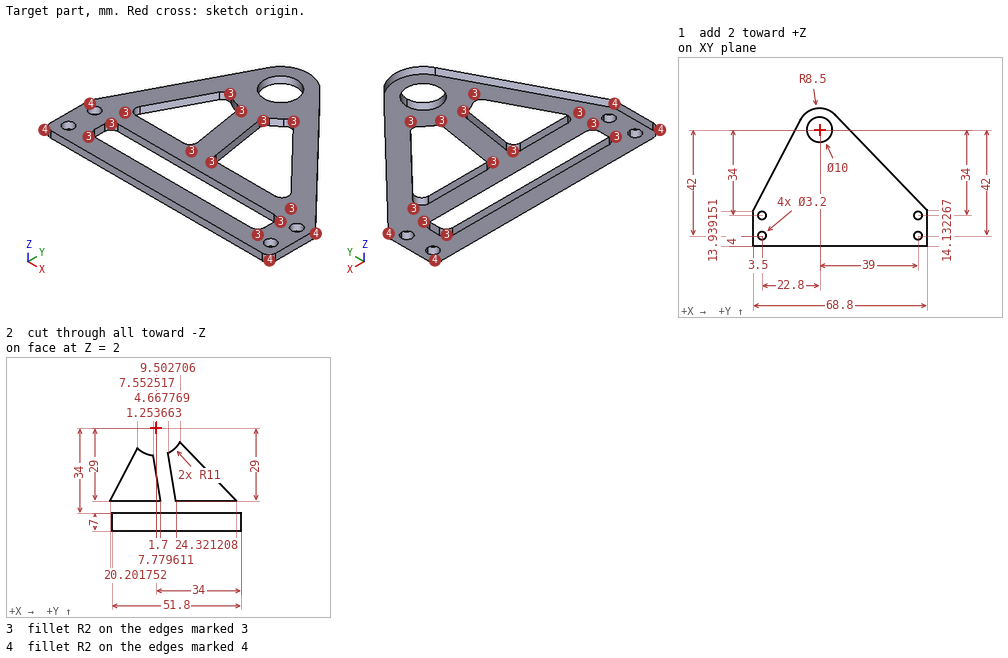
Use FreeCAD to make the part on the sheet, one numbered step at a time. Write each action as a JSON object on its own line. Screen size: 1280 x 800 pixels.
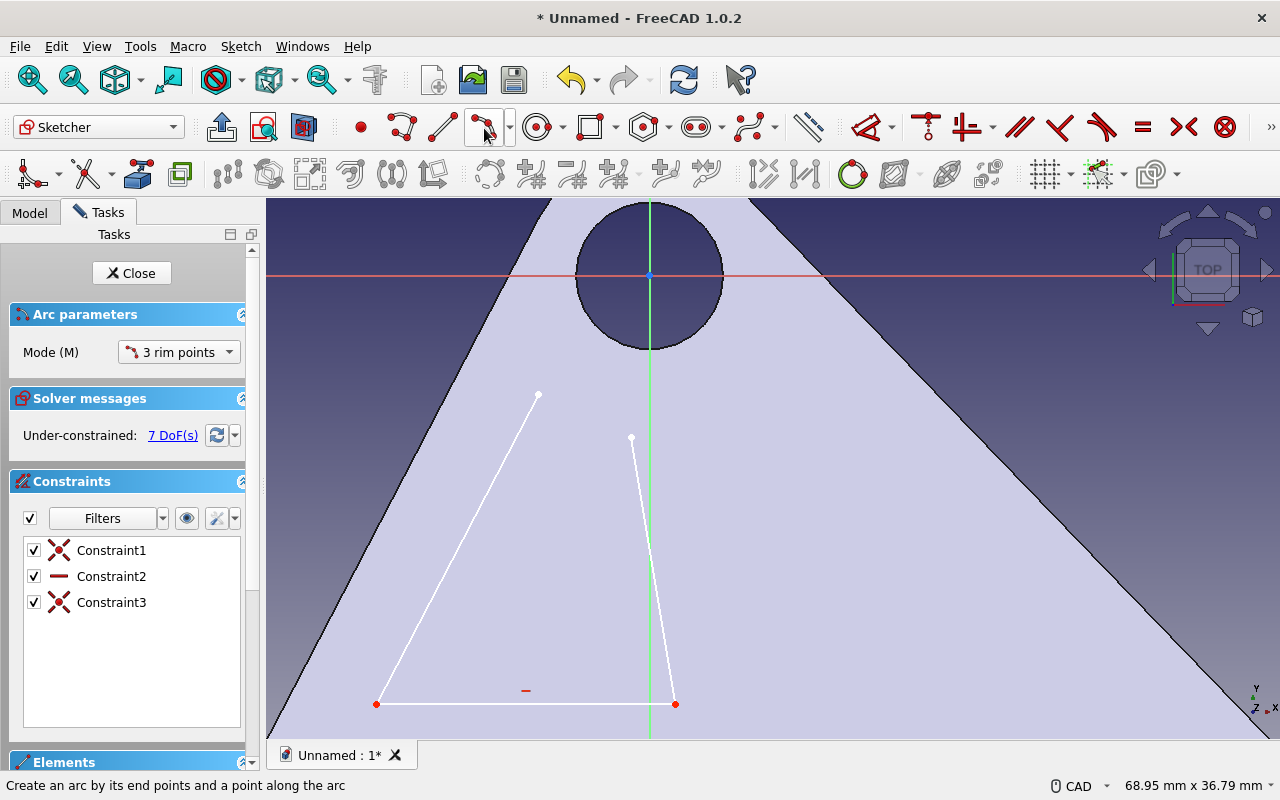
{"action": "left_click", "coordinate": [631, 438]}
{"action": "left_click", "coordinate": [539, 395]}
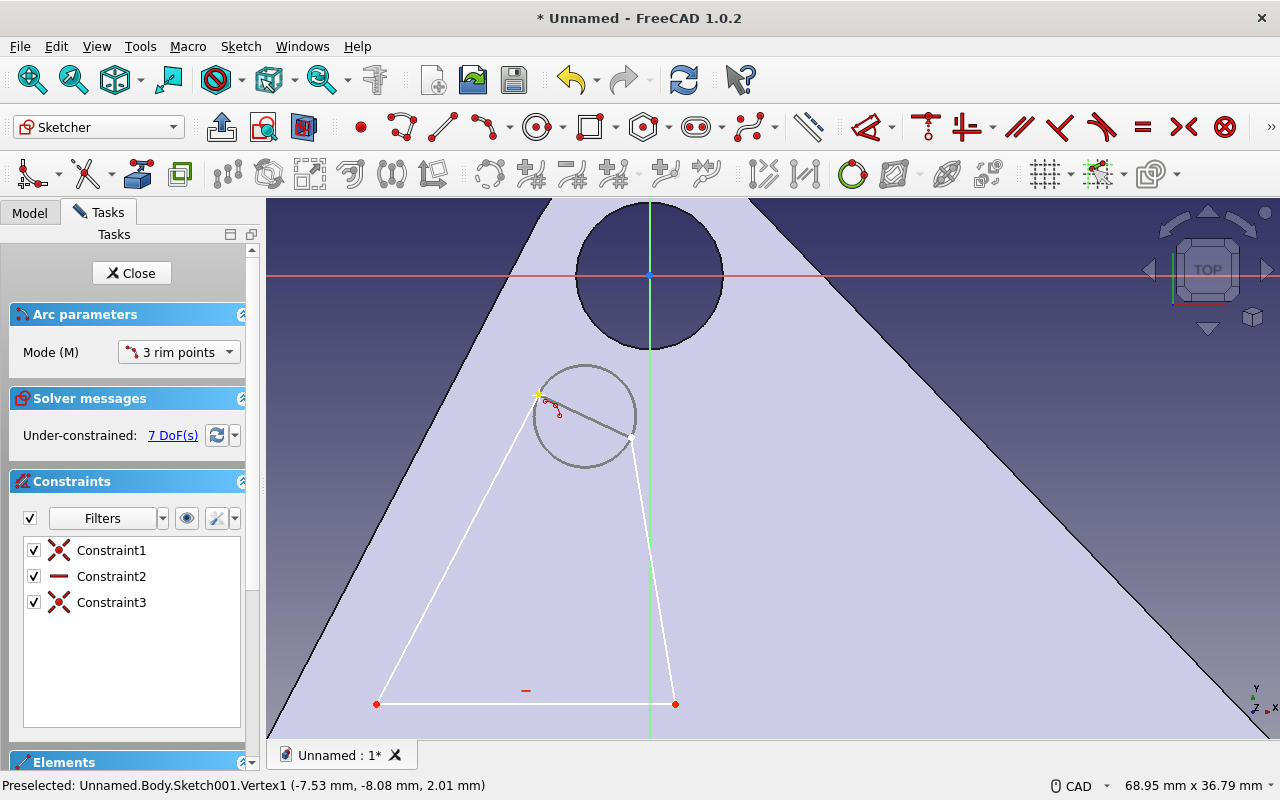
{"action": "scroll", "coordinate": [581, 423], "scroll_direction": "up", "scroll_amount": 4}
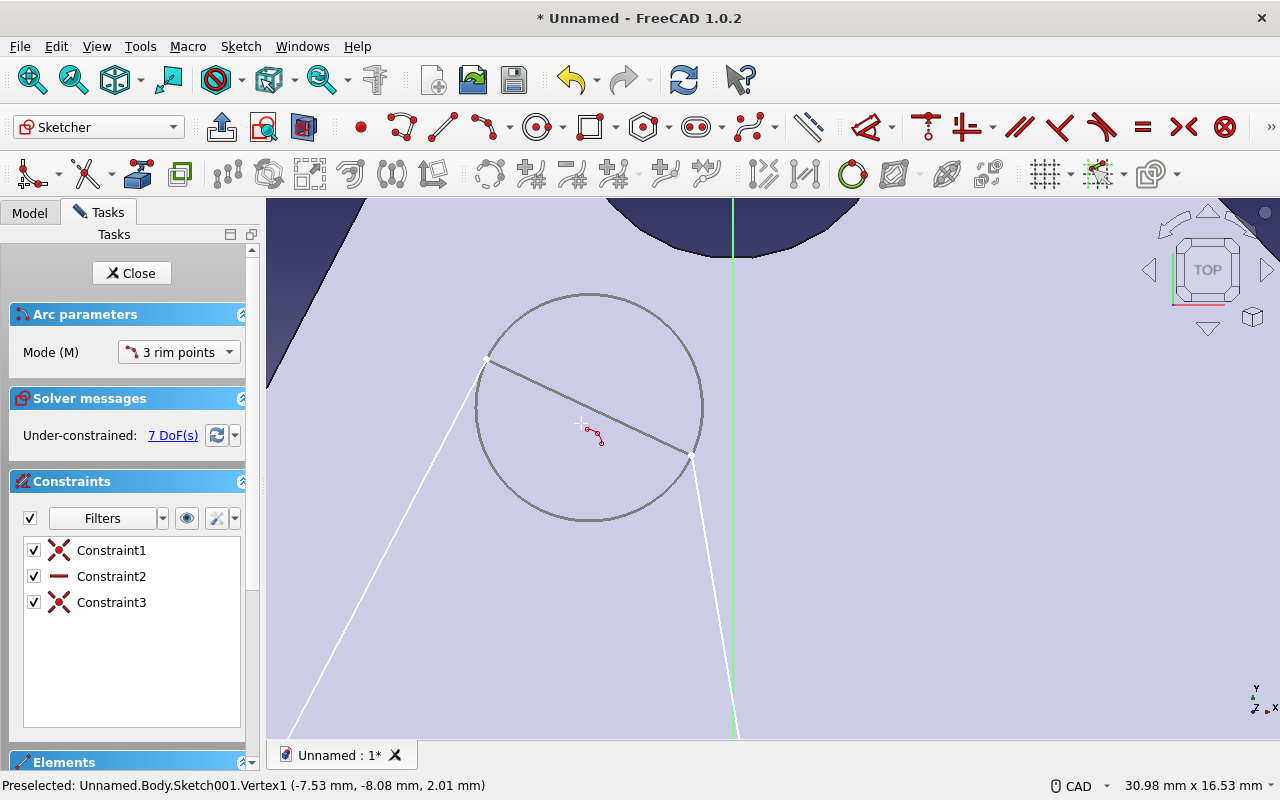
{"action": "left_click", "coordinate": [581, 421]}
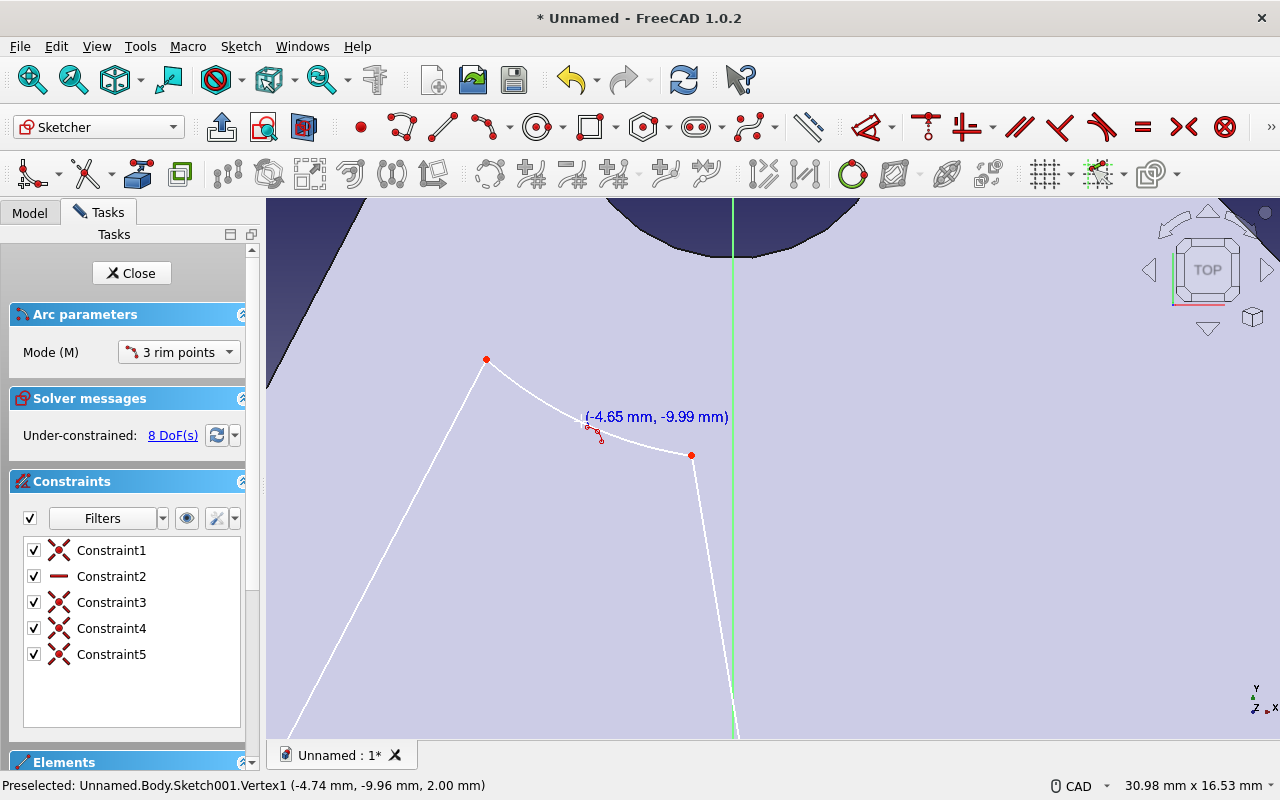
{"action": "left_click", "coordinate": [402, 128]}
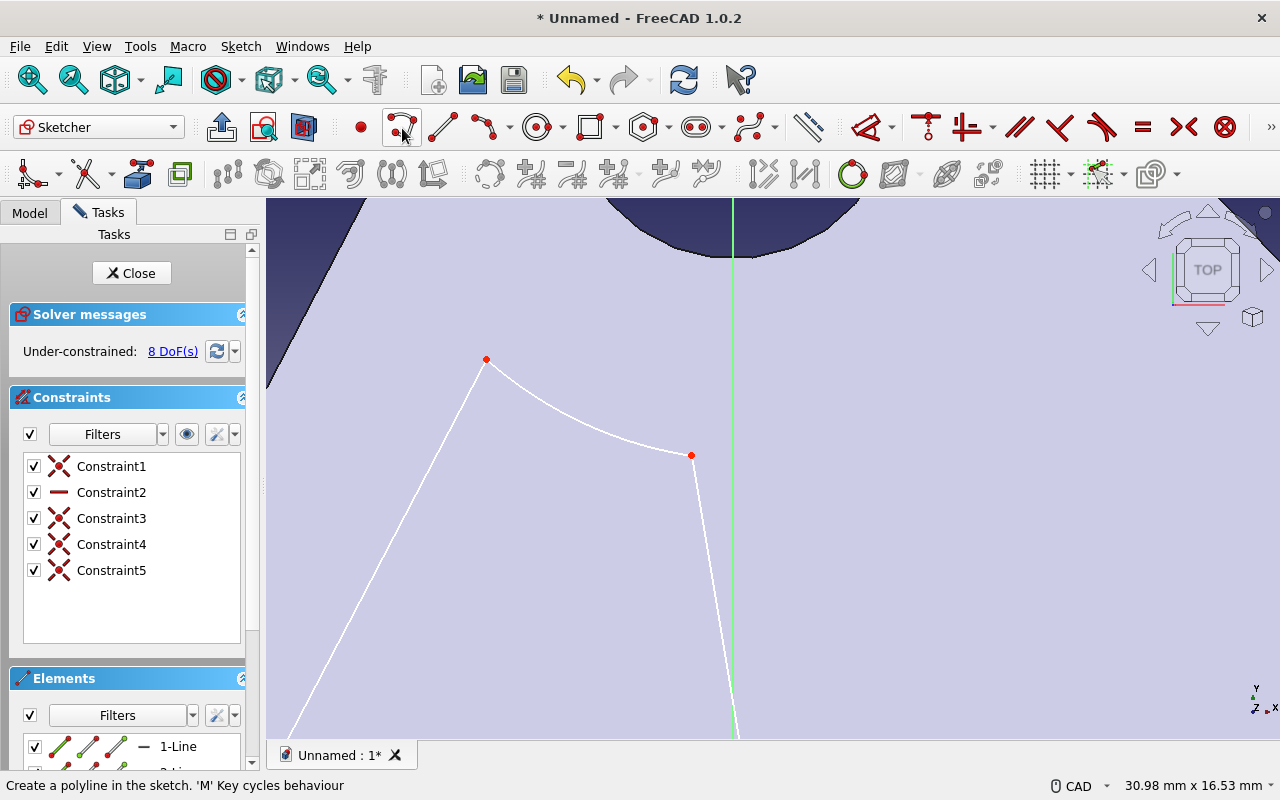
{"action": "scroll", "coordinate": [612, 371], "scroll_direction": "down", "scroll_amount": 7}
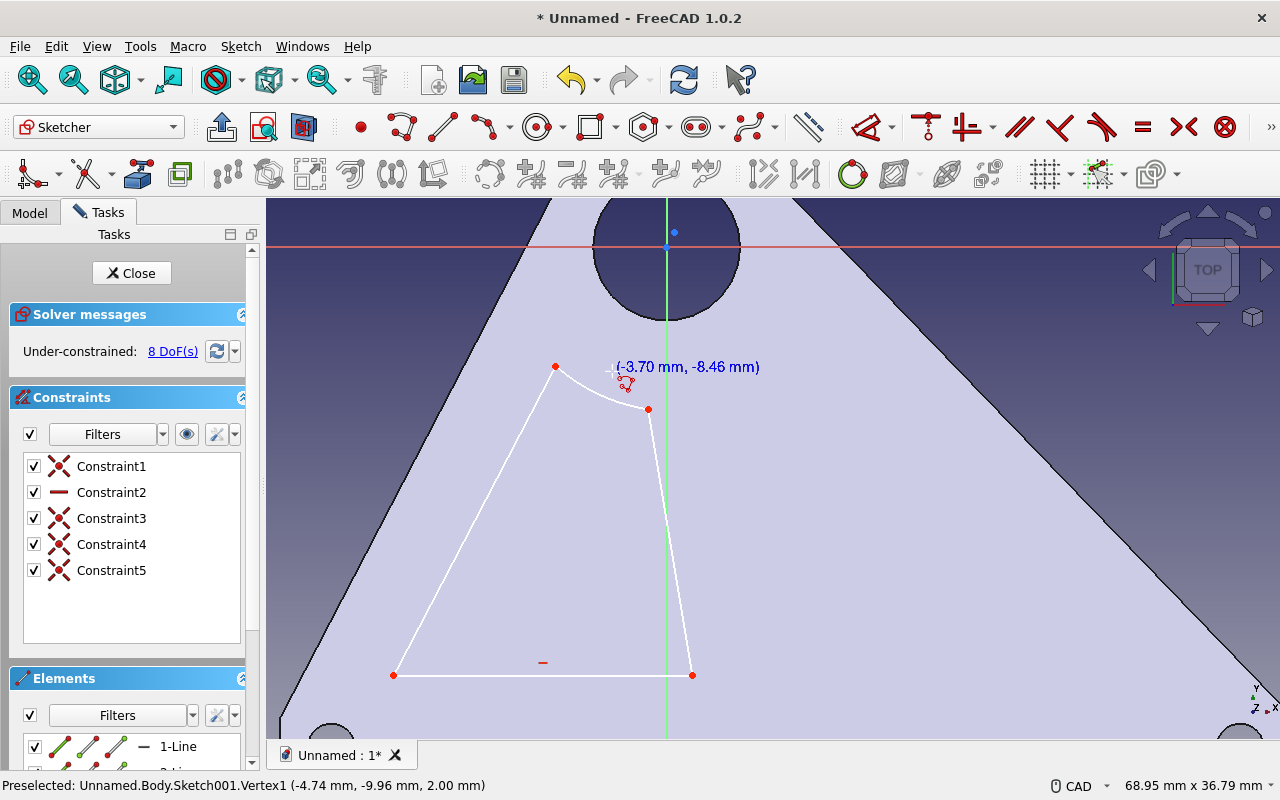
{"action": "left_click", "coordinate": [680, 384]}
{"action": "left_click", "coordinate": [705, 537]}
{"action": "left_click", "coordinate": [901, 537]}
{"action": "left_click", "coordinate": [719, 348]}
{"action": "right_click", "coordinate": [719, 348]}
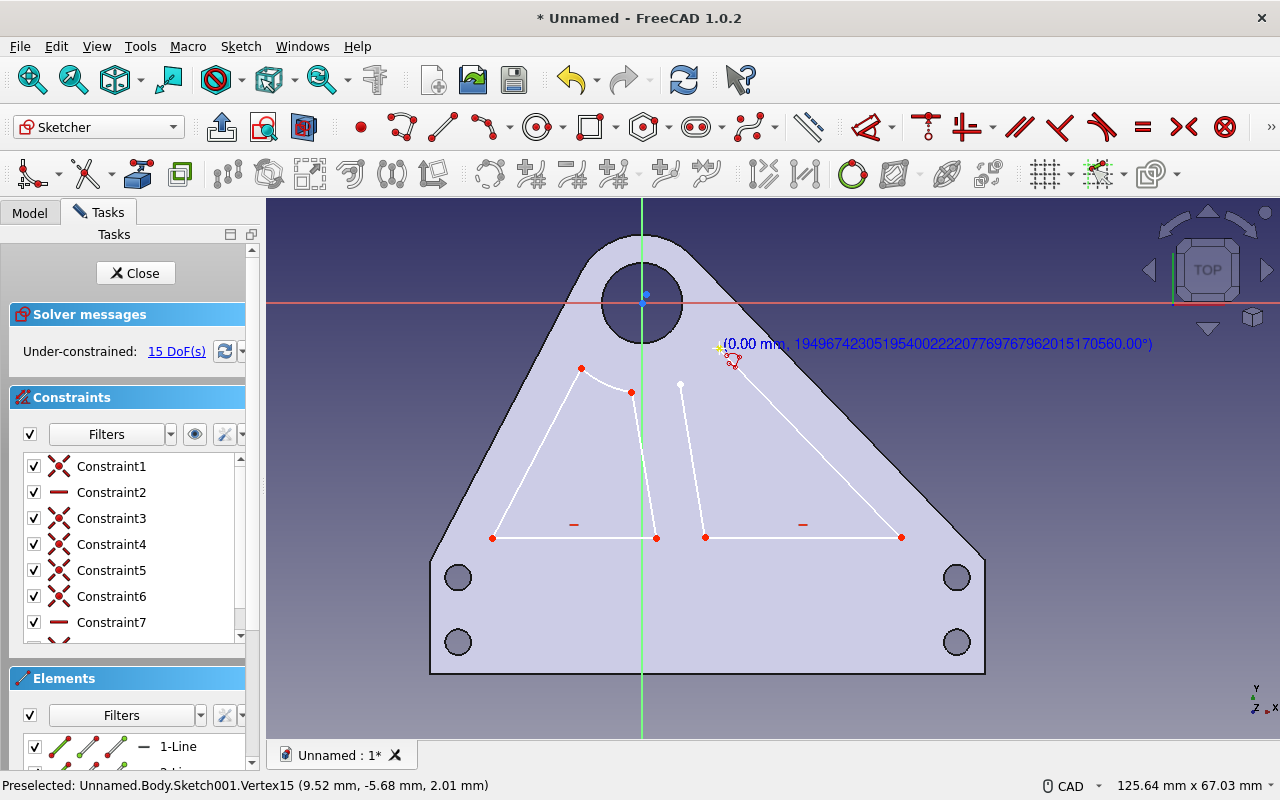
{"action": "key", "text": "g 3 a"}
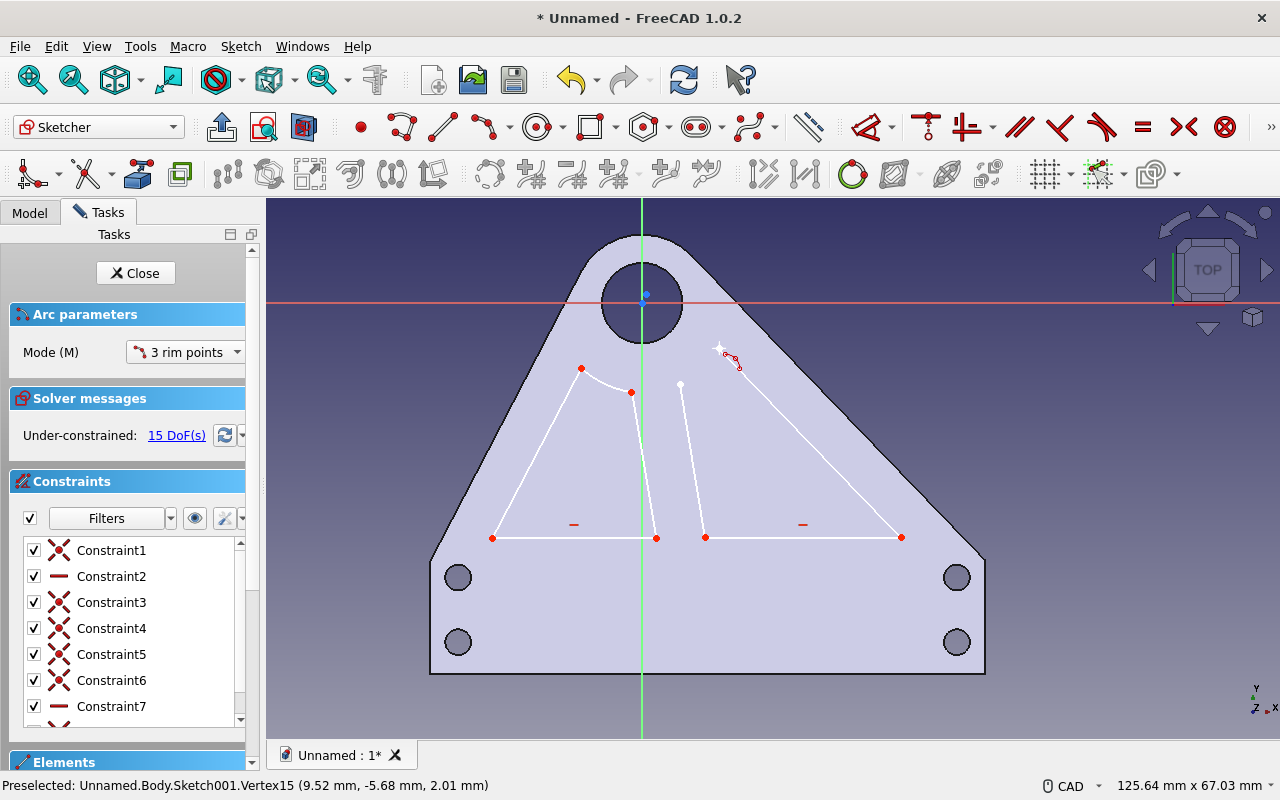
{"action": "left_click", "coordinate": [719, 349]}
{"action": "left_click", "coordinate": [680, 385]}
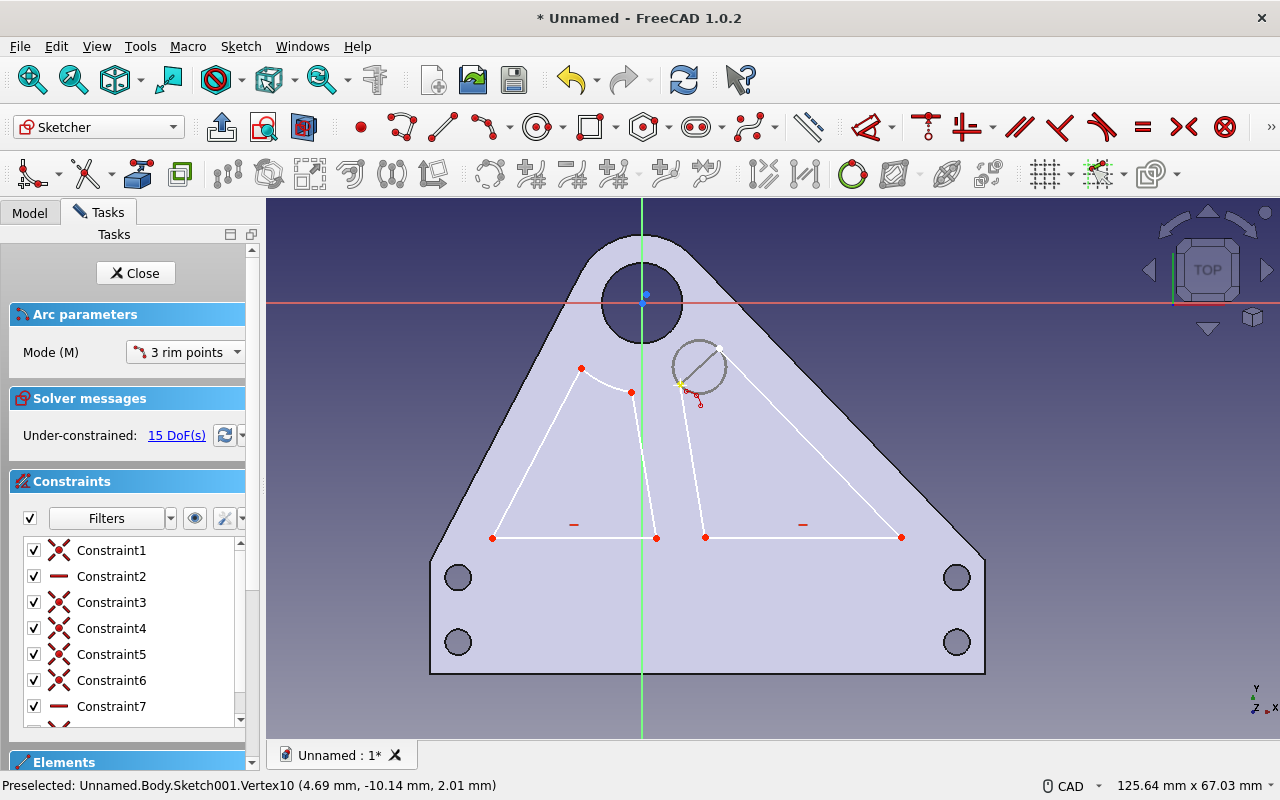
{"action": "scroll", "coordinate": [702, 369], "scroll_direction": "up", "scroll_amount": 7}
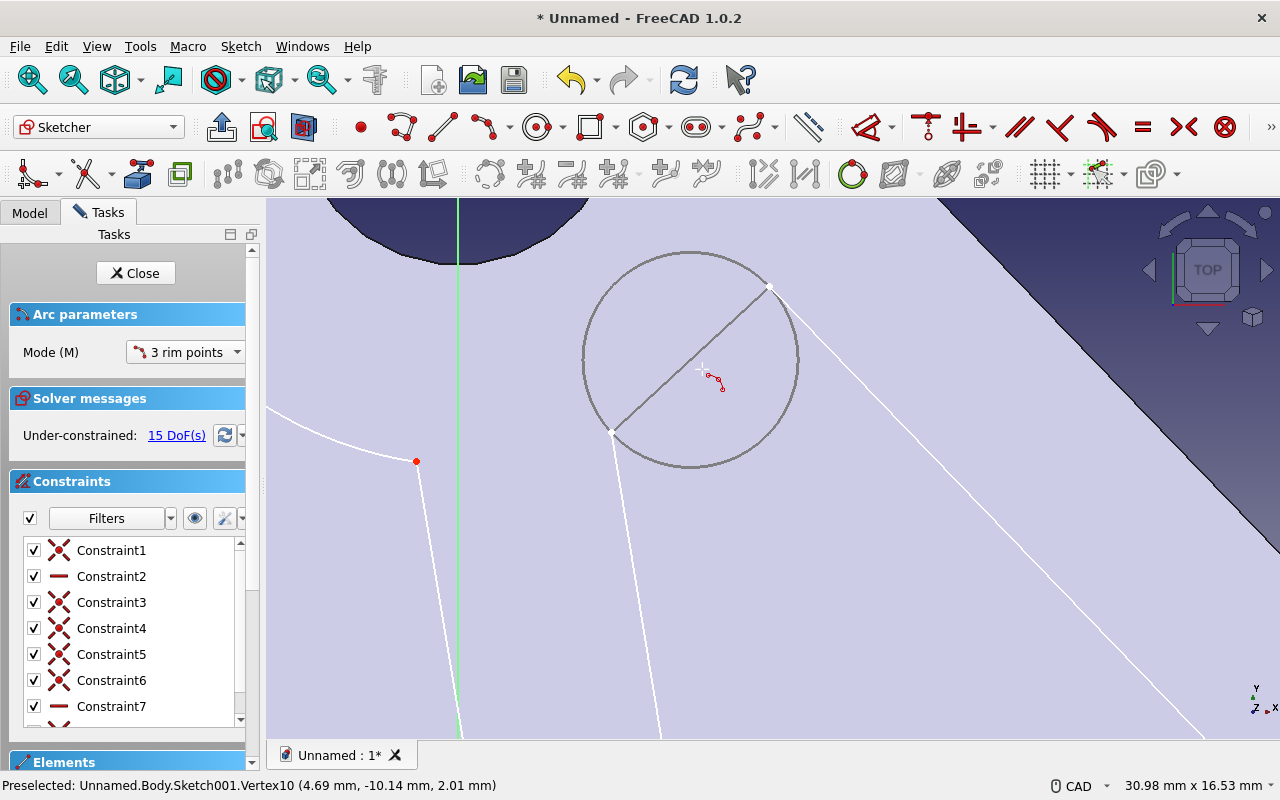
{"action": "left_click", "coordinate": [701, 367]}